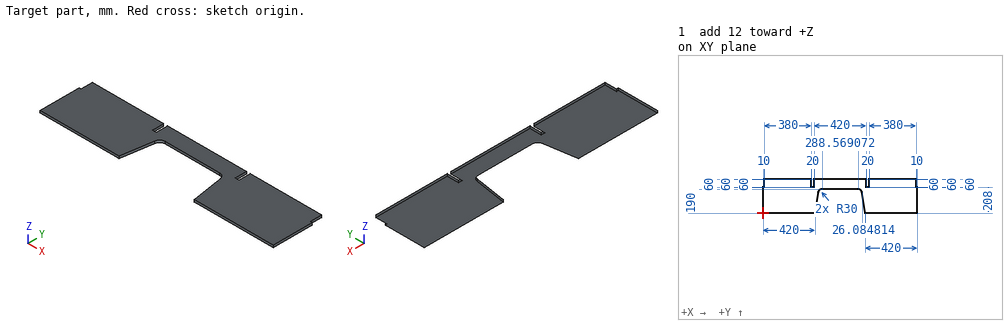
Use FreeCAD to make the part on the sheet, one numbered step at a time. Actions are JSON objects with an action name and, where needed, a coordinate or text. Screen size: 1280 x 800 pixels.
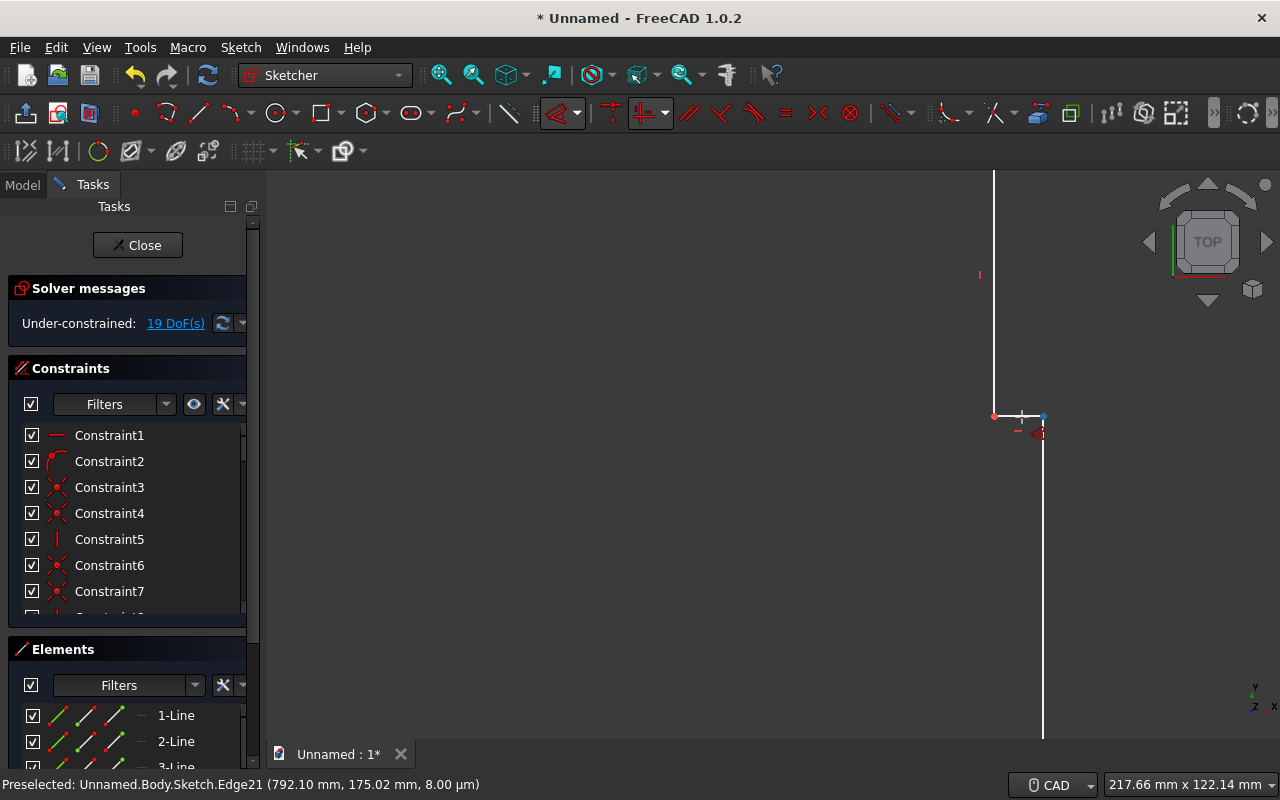
{"action": "left_click", "coordinate": [1019, 416]}
{"action": "left_click", "coordinate": [1019, 382]}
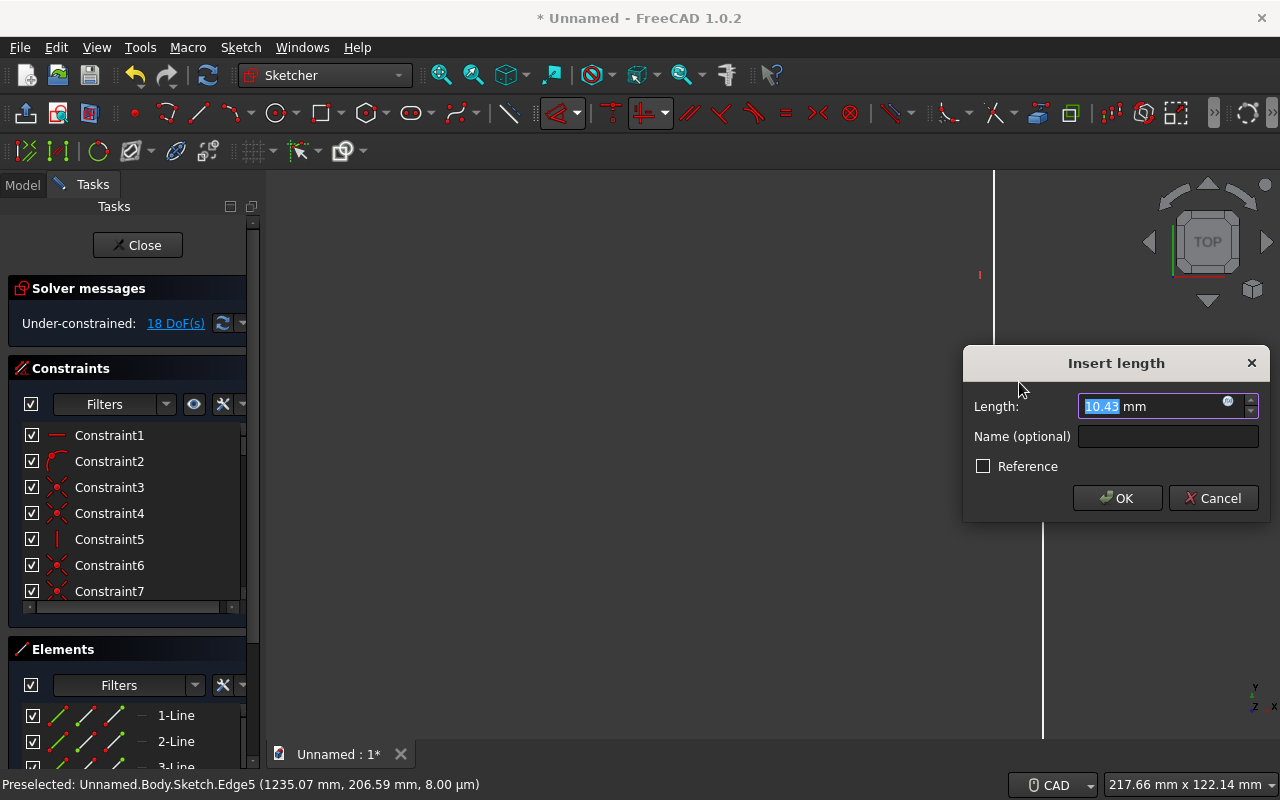
{"action": "type", "text": "10"}
{"action": "key", "text": "Return"}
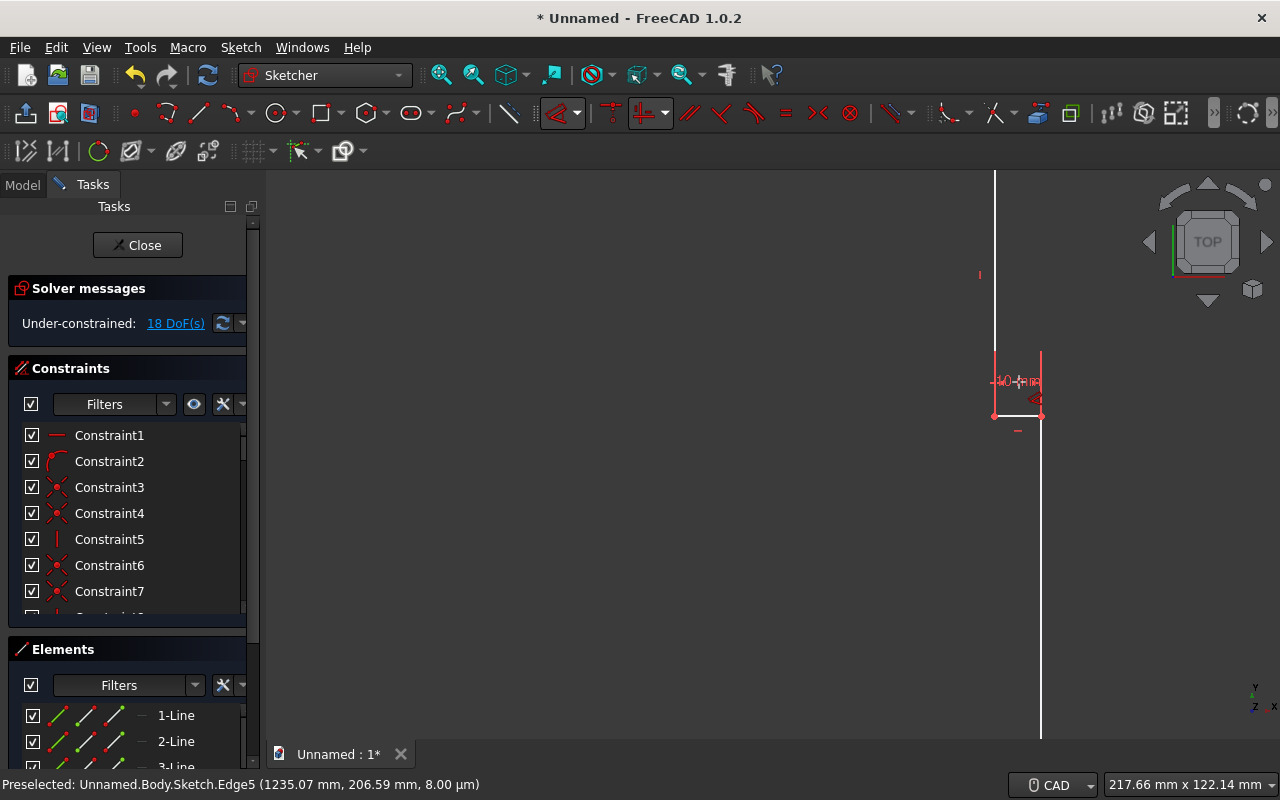
{"action": "scroll", "coordinate": [1022, 417], "scroll_direction": "down", "scroll_amount": 11}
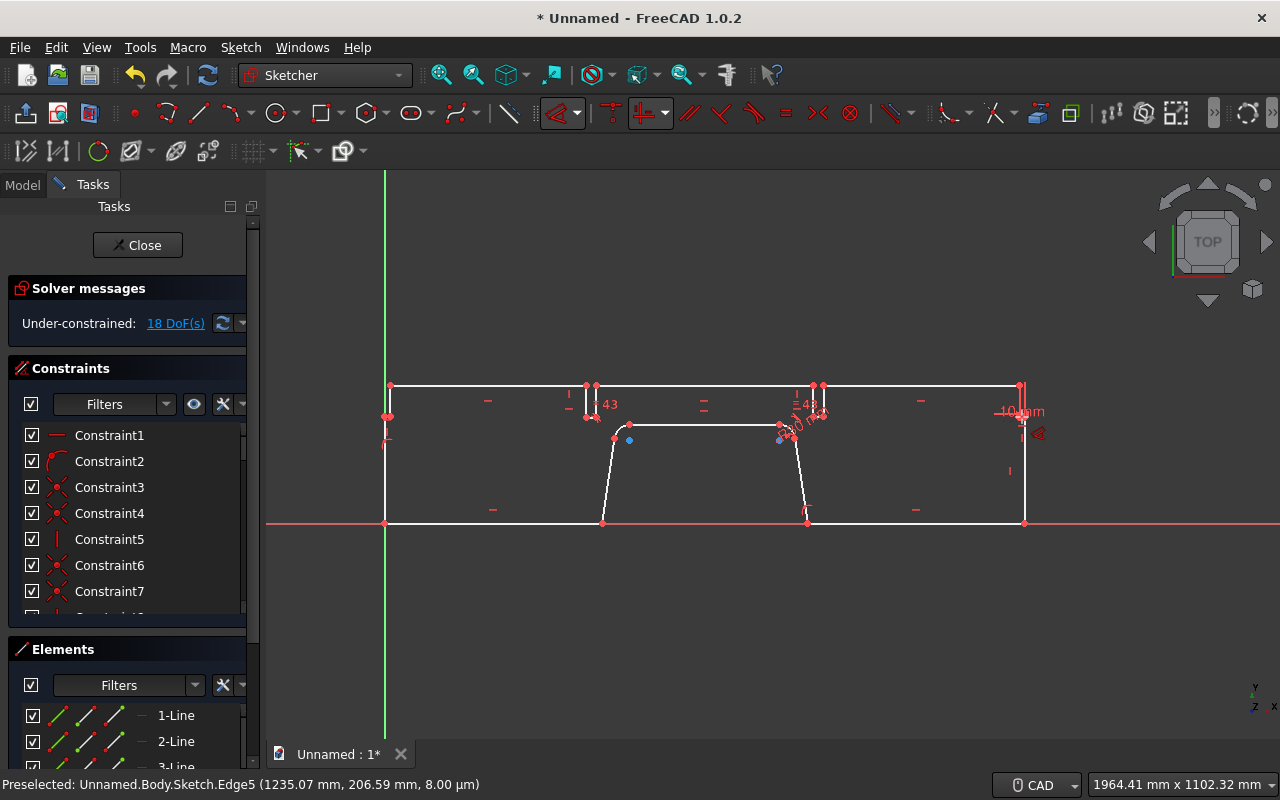
{"action": "scroll", "coordinate": [1020, 408], "scroll_direction": "up", "scroll_amount": 2}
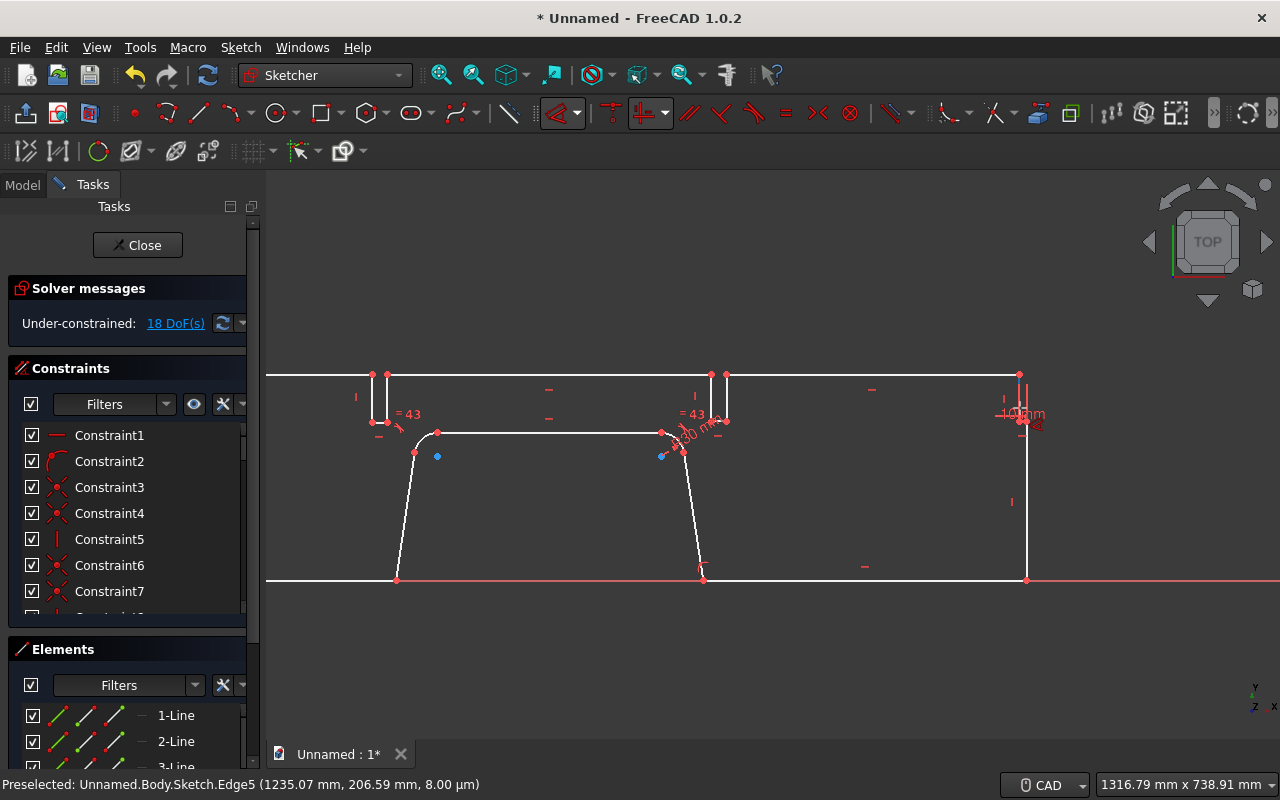
{"action": "left_click", "coordinate": [1019, 408]}
{"action": "left_click", "coordinate": [1053, 387]}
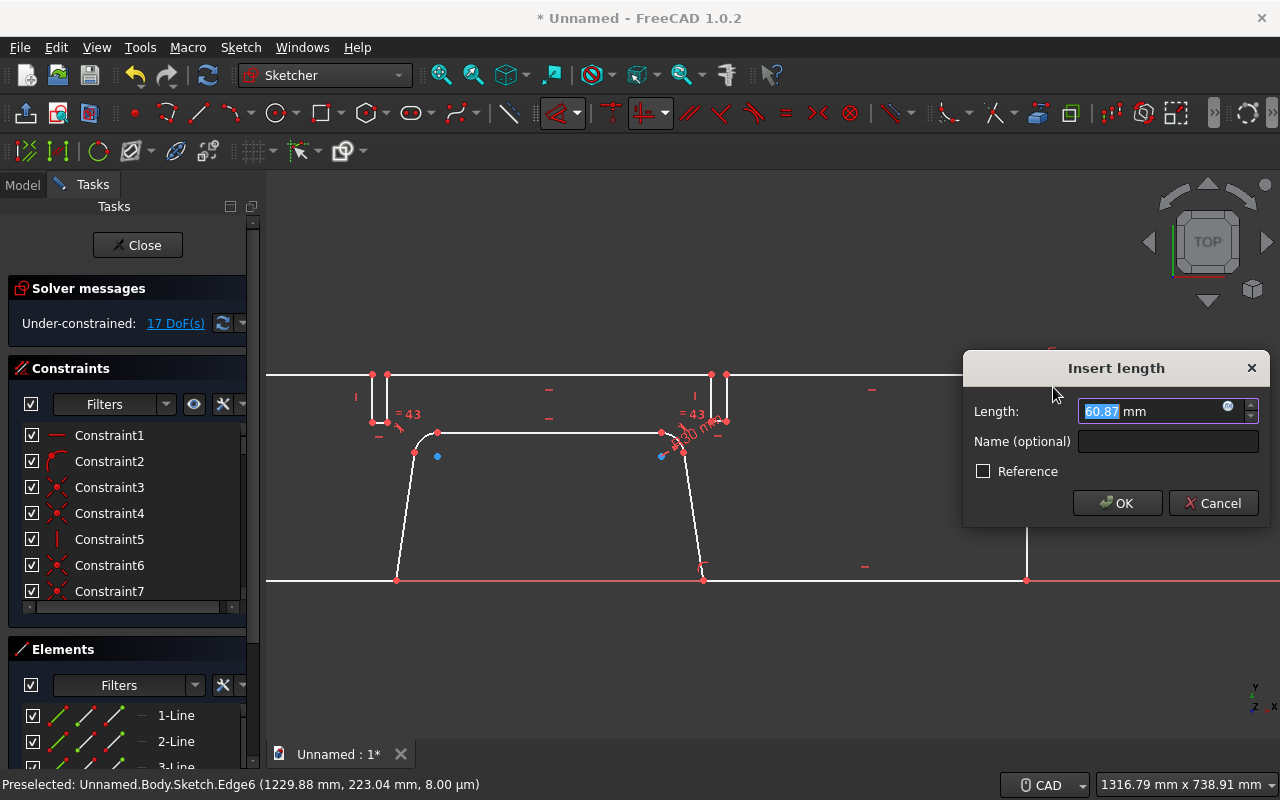
{"action": "type", "text": "60"}
{"action": "key", "text": "Return"}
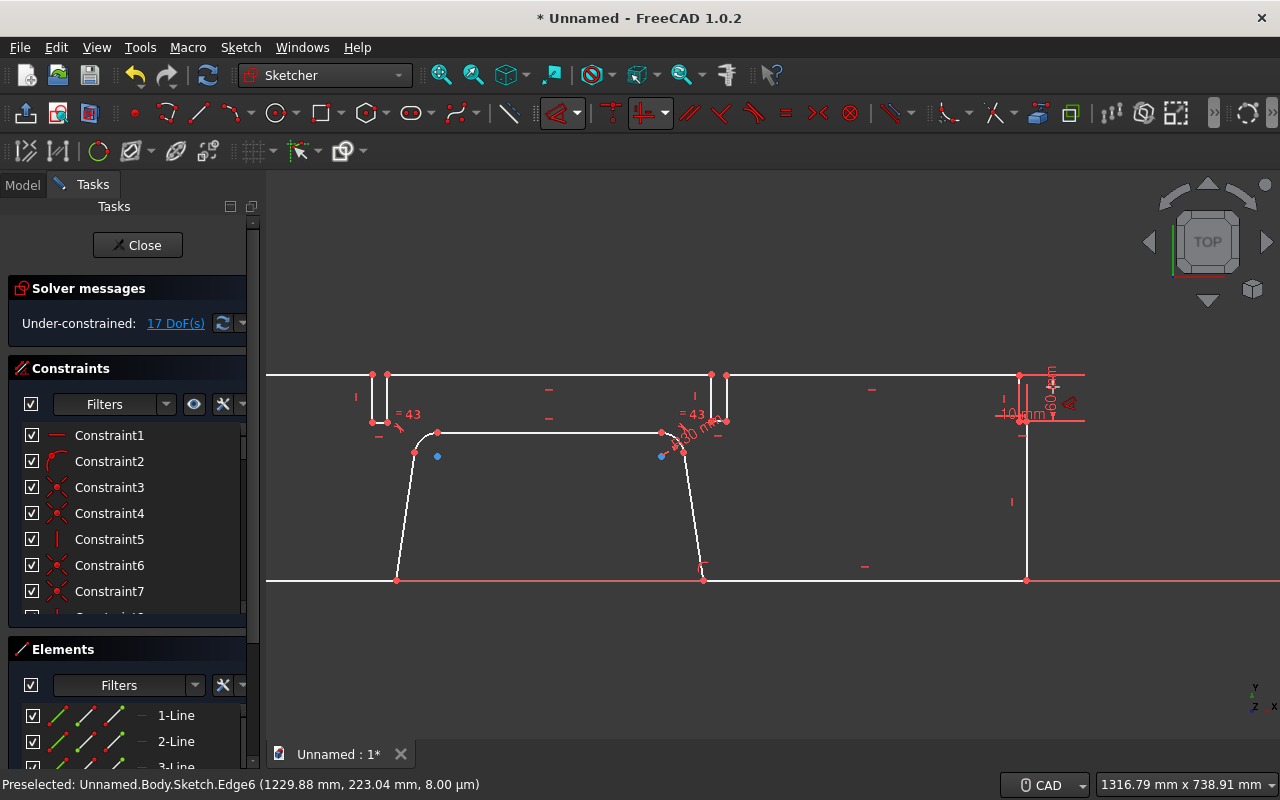
{"action": "left_click", "coordinate": [727, 389]}
{"action": "left_click", "coordinate": [761, 398]}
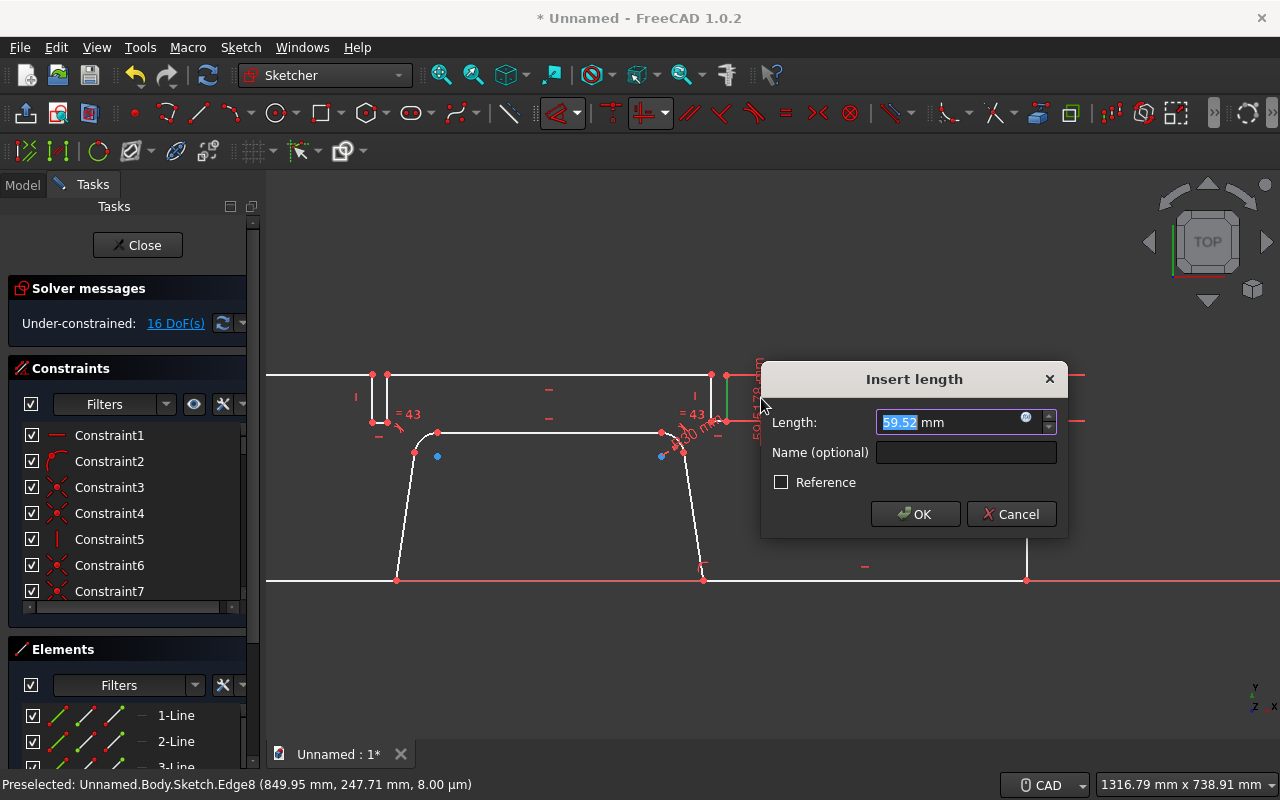
{"action": "type", "text": "60"}
{"action": "key", "text": "Return"}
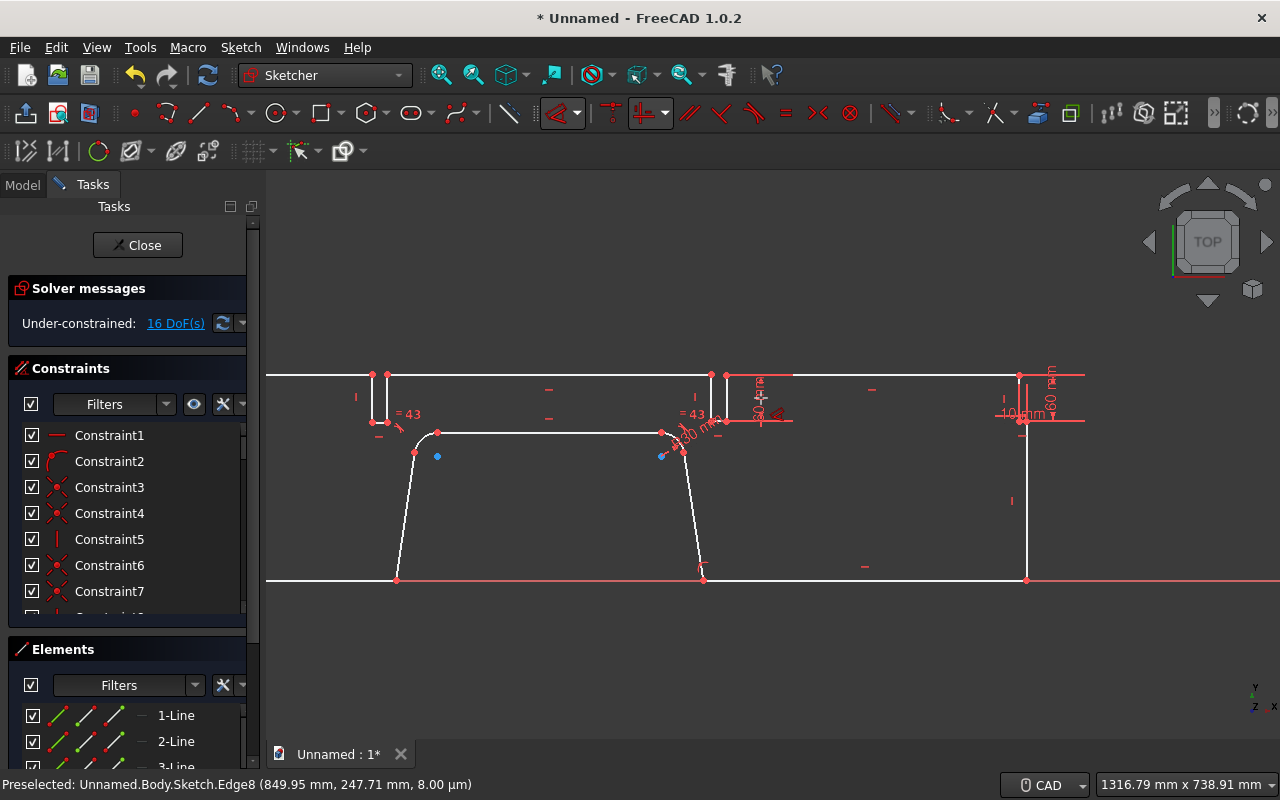
{"action": "scroll", "coordinate": [719, 421], "scroll_direction": "up", "scroll_amount": 5}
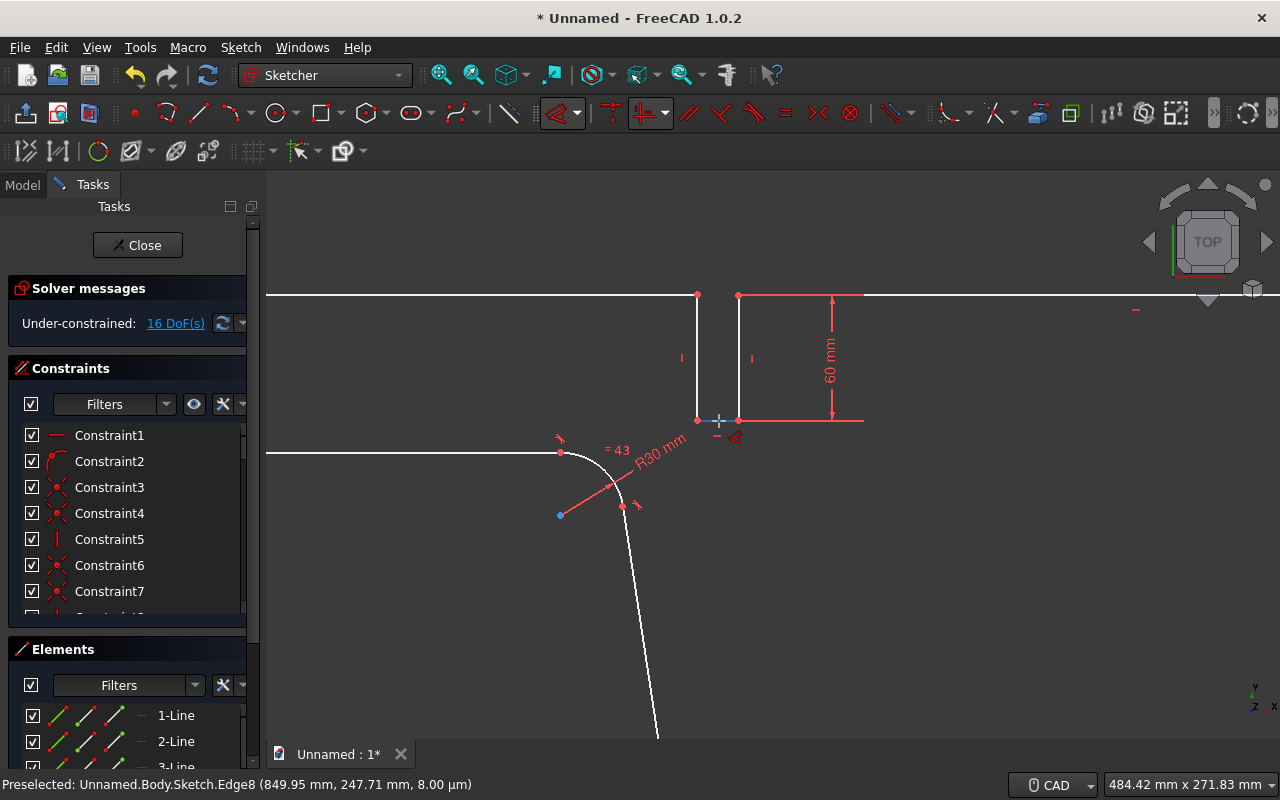
{"action": "left_click", "coordinate": [718, 421]}
{"action": "left_click", "coordinate": [718, 387]}